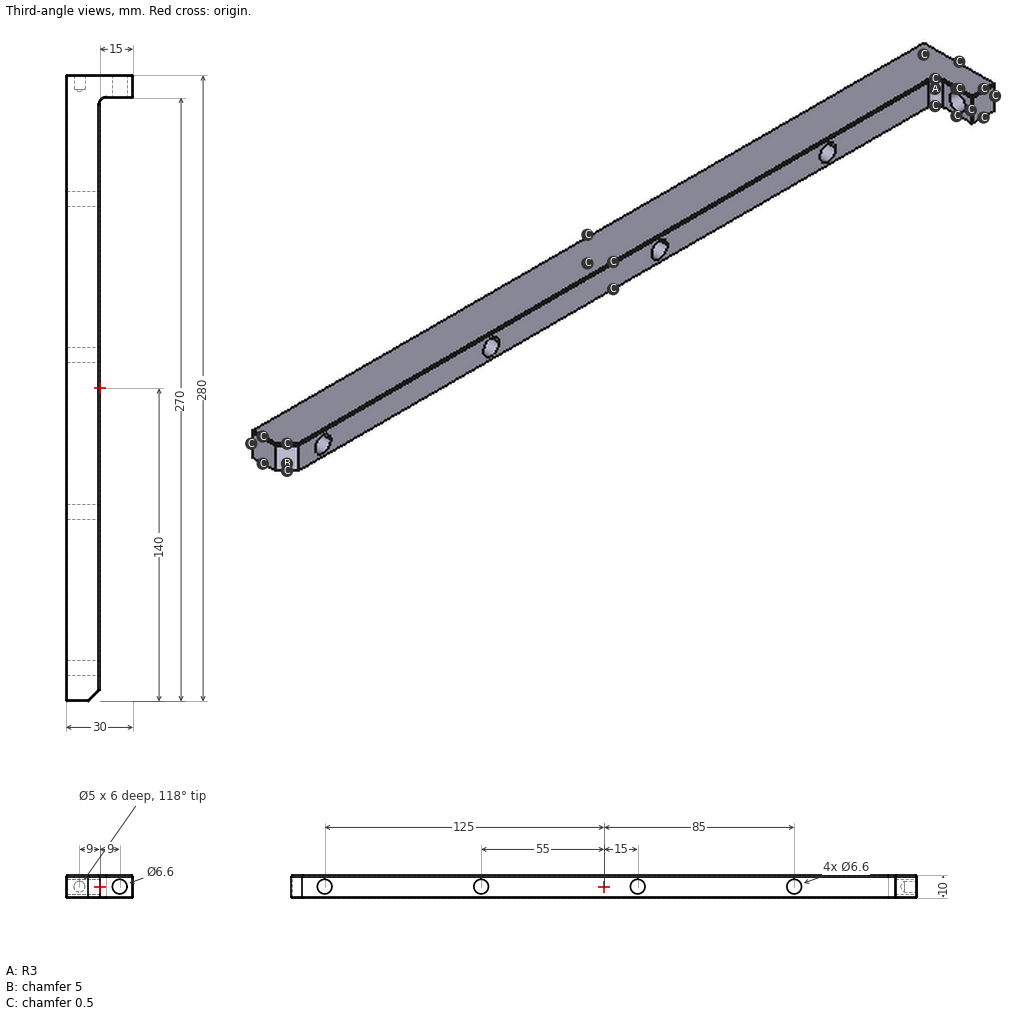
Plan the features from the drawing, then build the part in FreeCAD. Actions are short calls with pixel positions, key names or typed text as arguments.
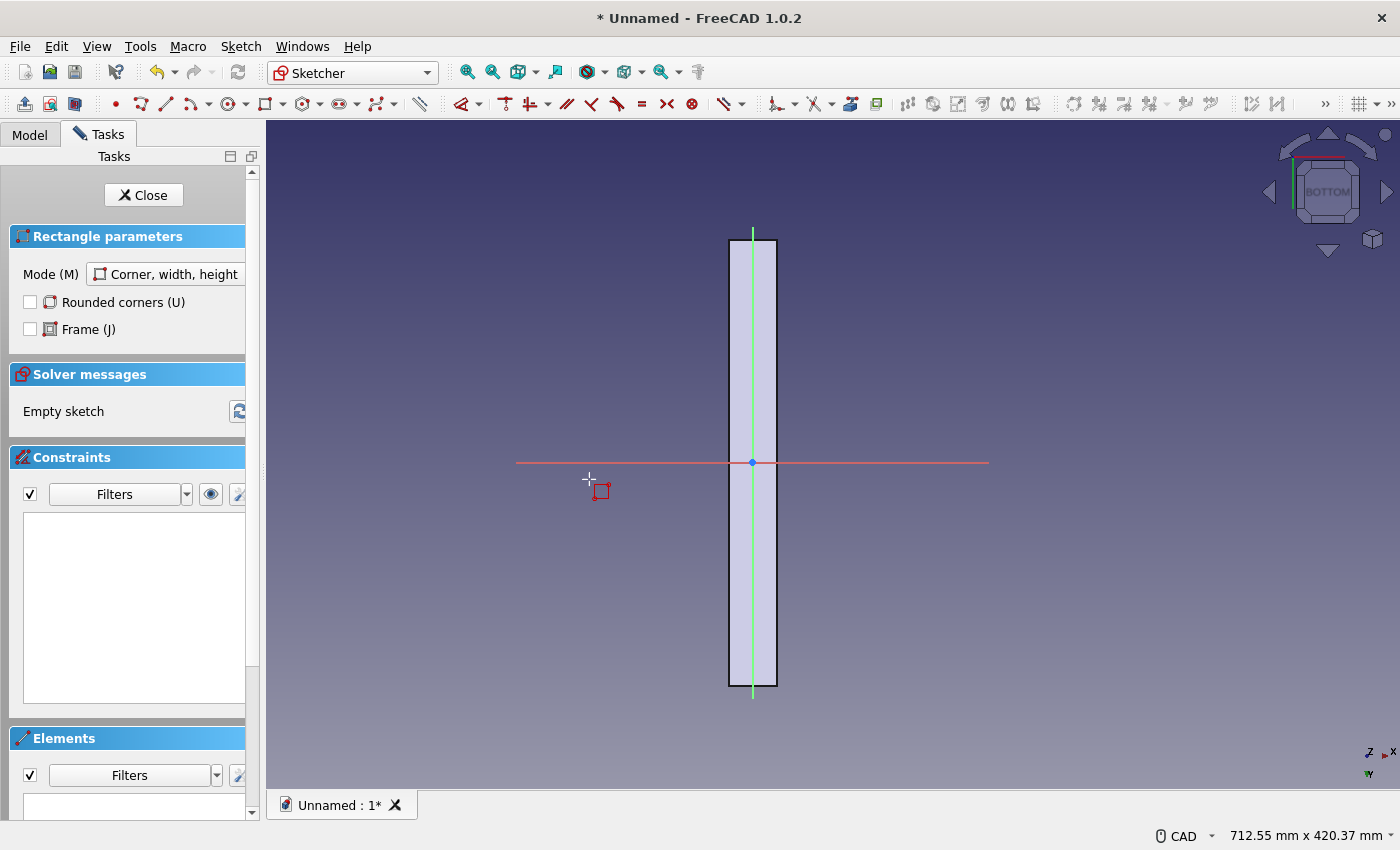
click(753, 240)
click(777, 670)
key(Escape)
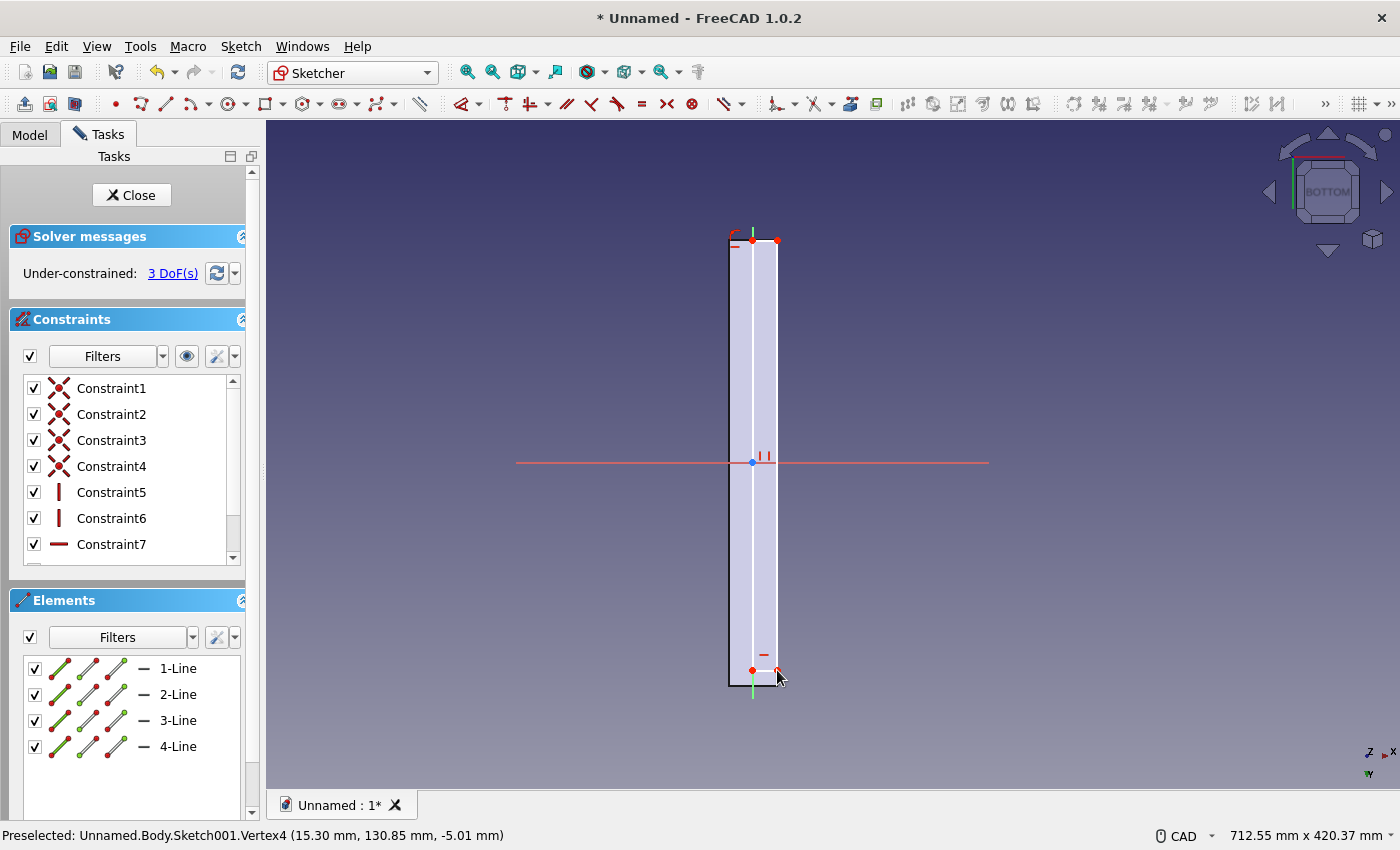
click(460, 104)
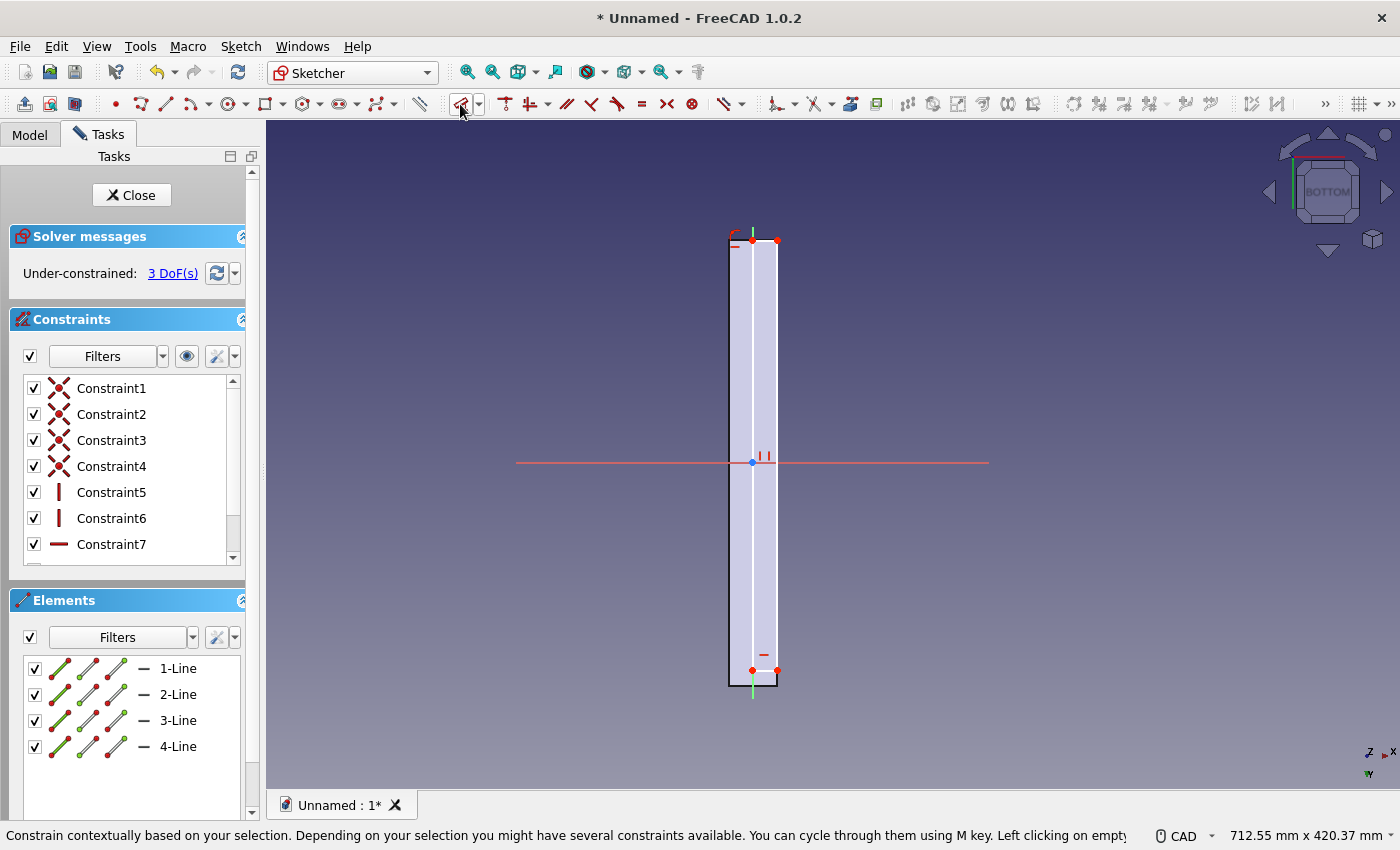
scroll(762, 671, up, 3)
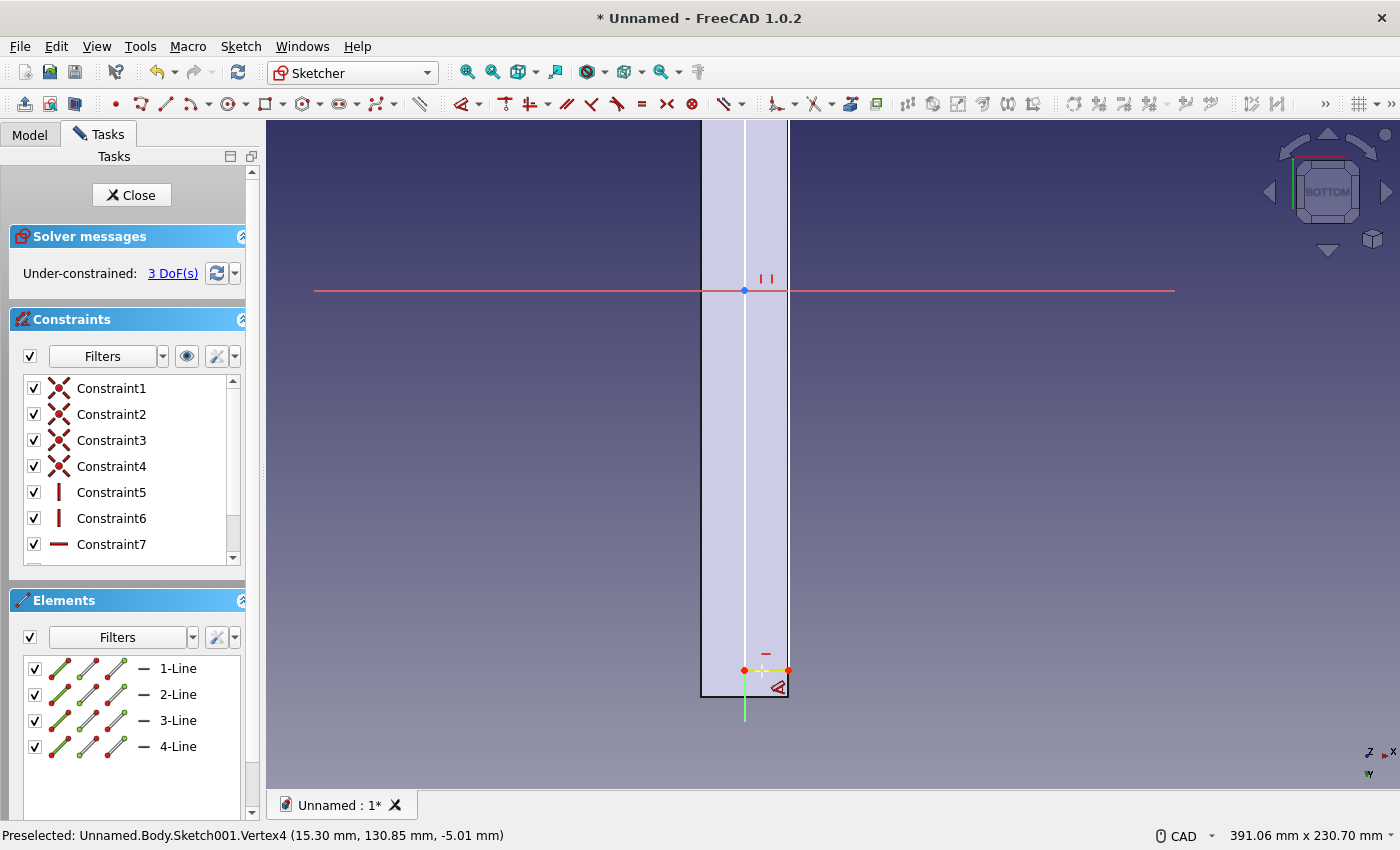
click(762, 670)
click(767, 704)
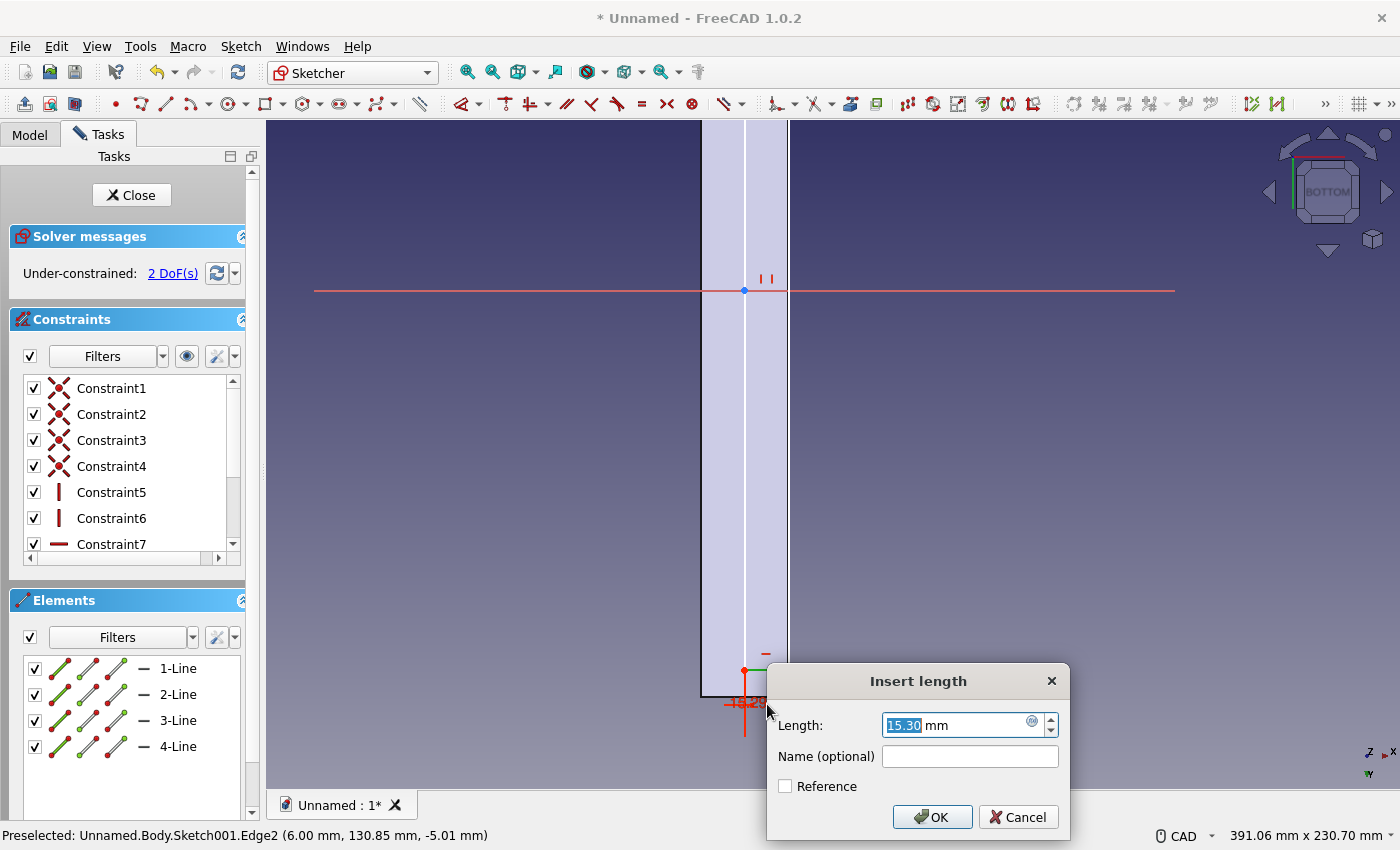
text(15)
key(Return)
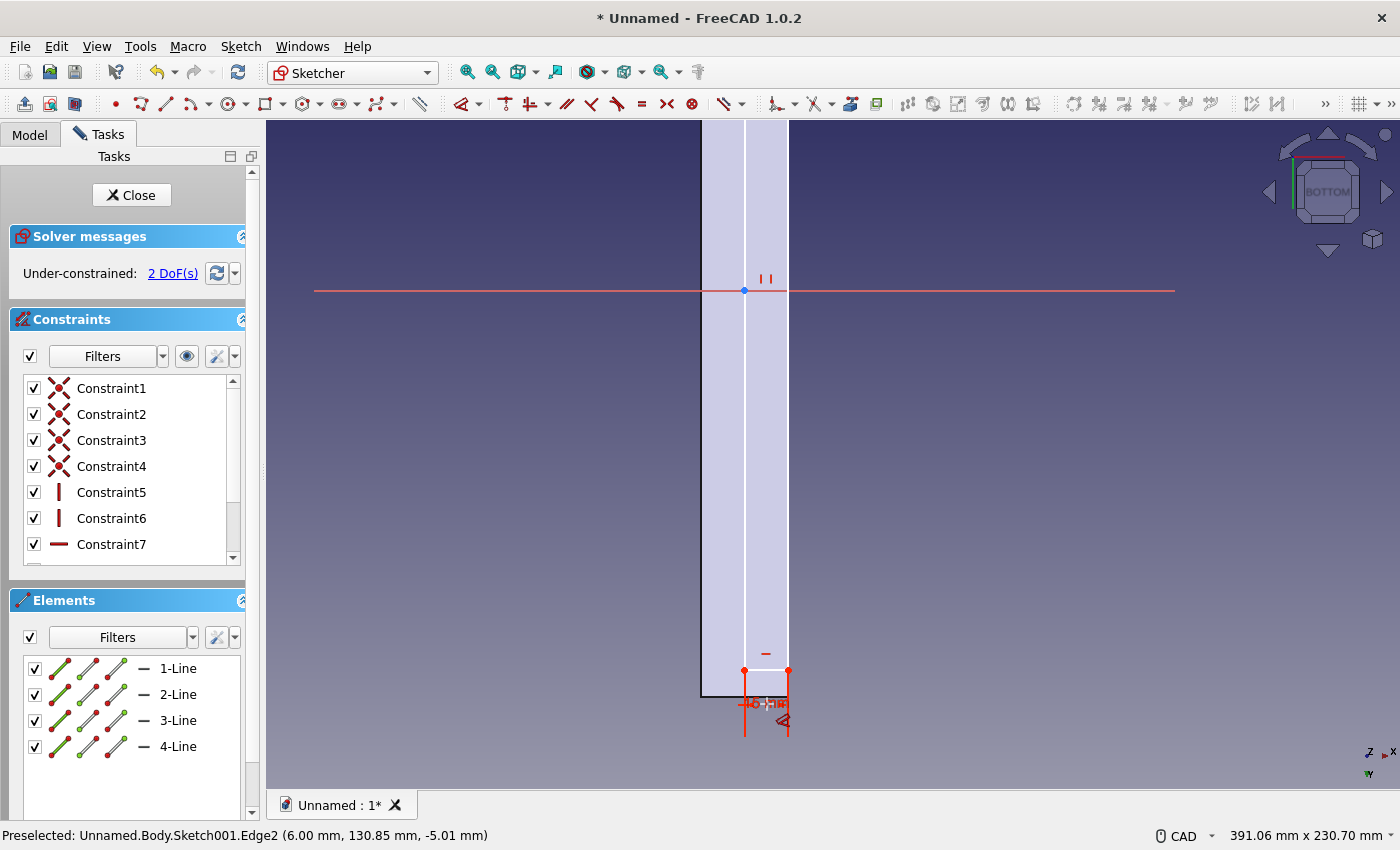
click(745, 435)
click(711, 409)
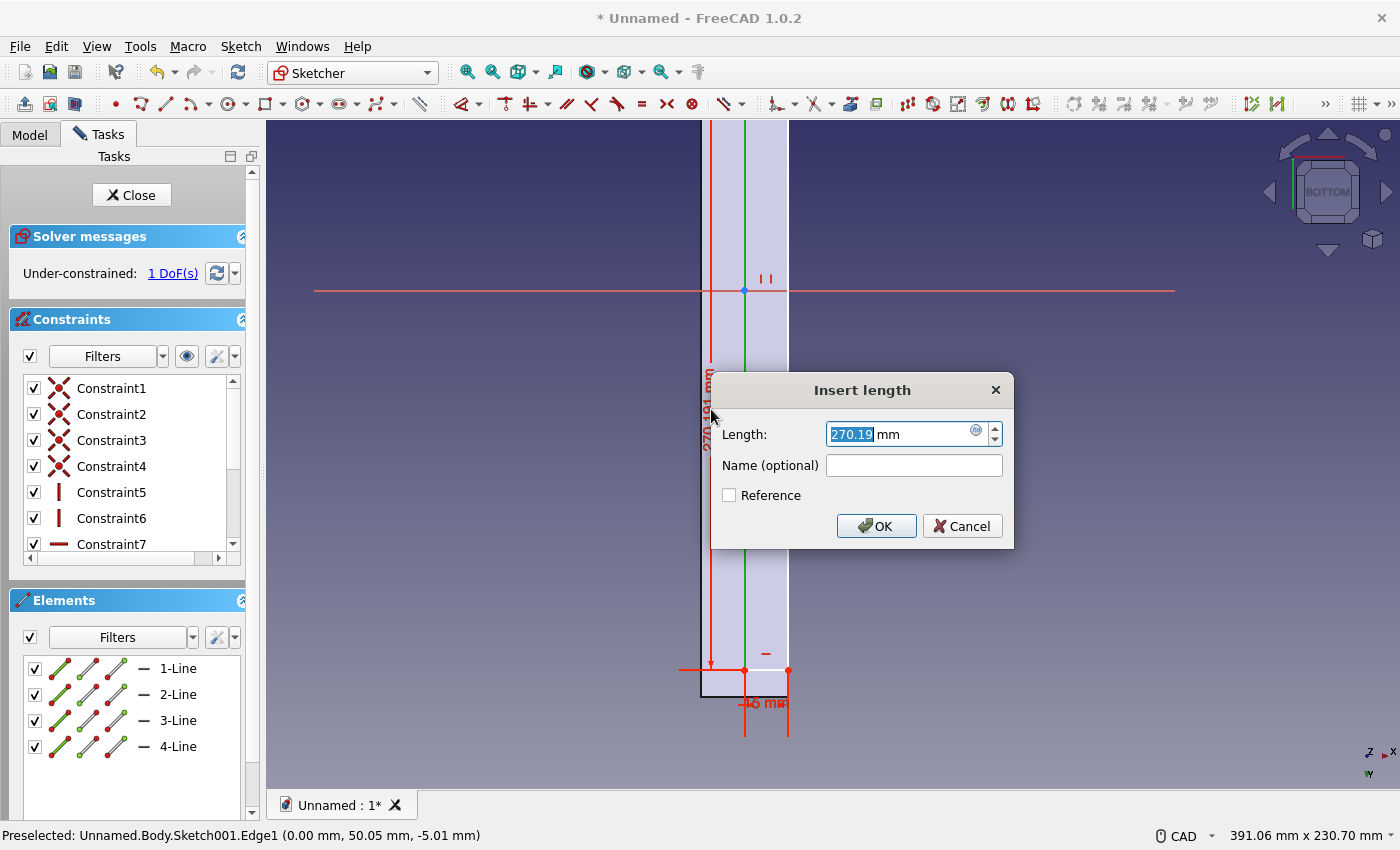
text(270)
key(Return)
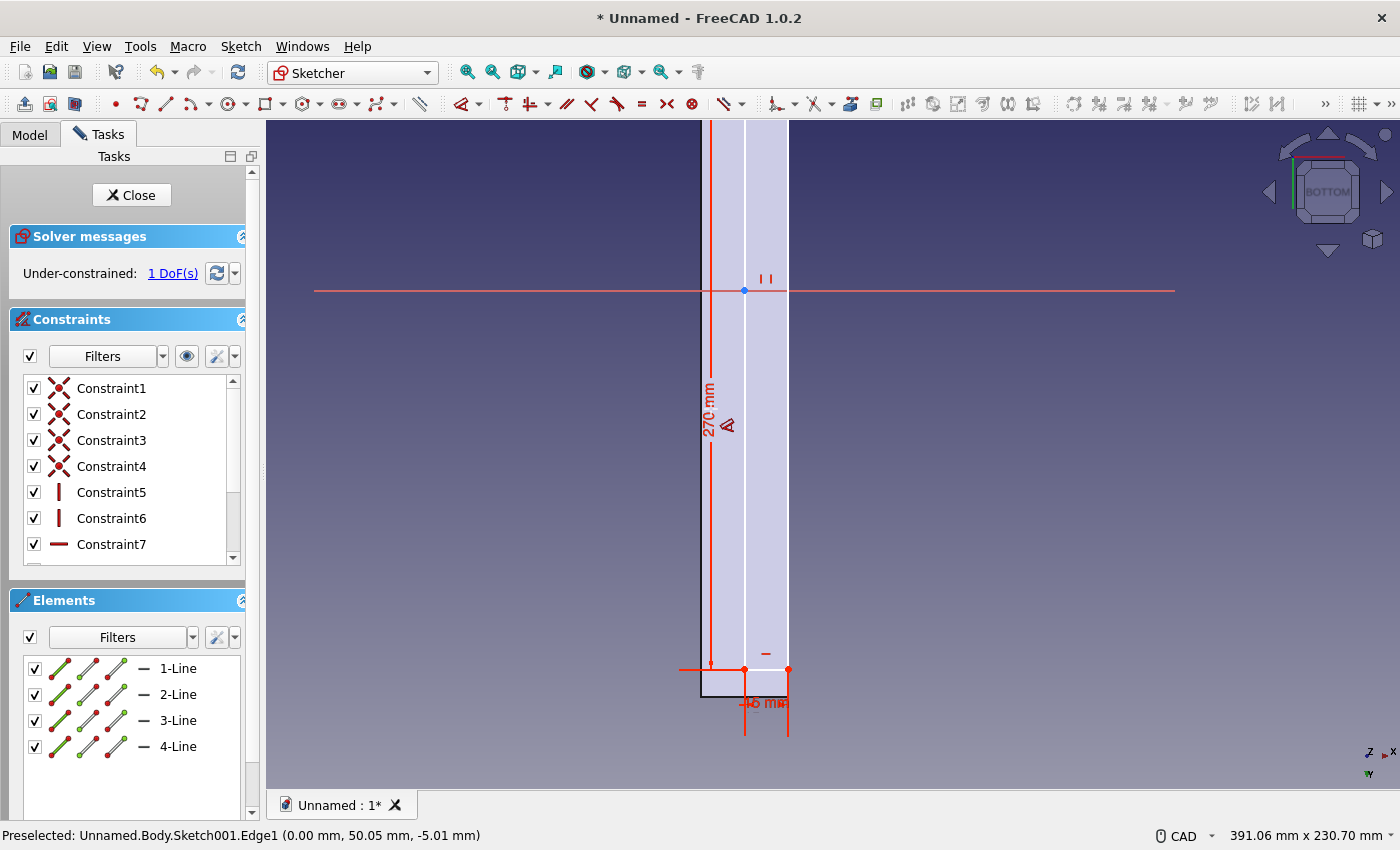
scroll(762, 671, down, 3)